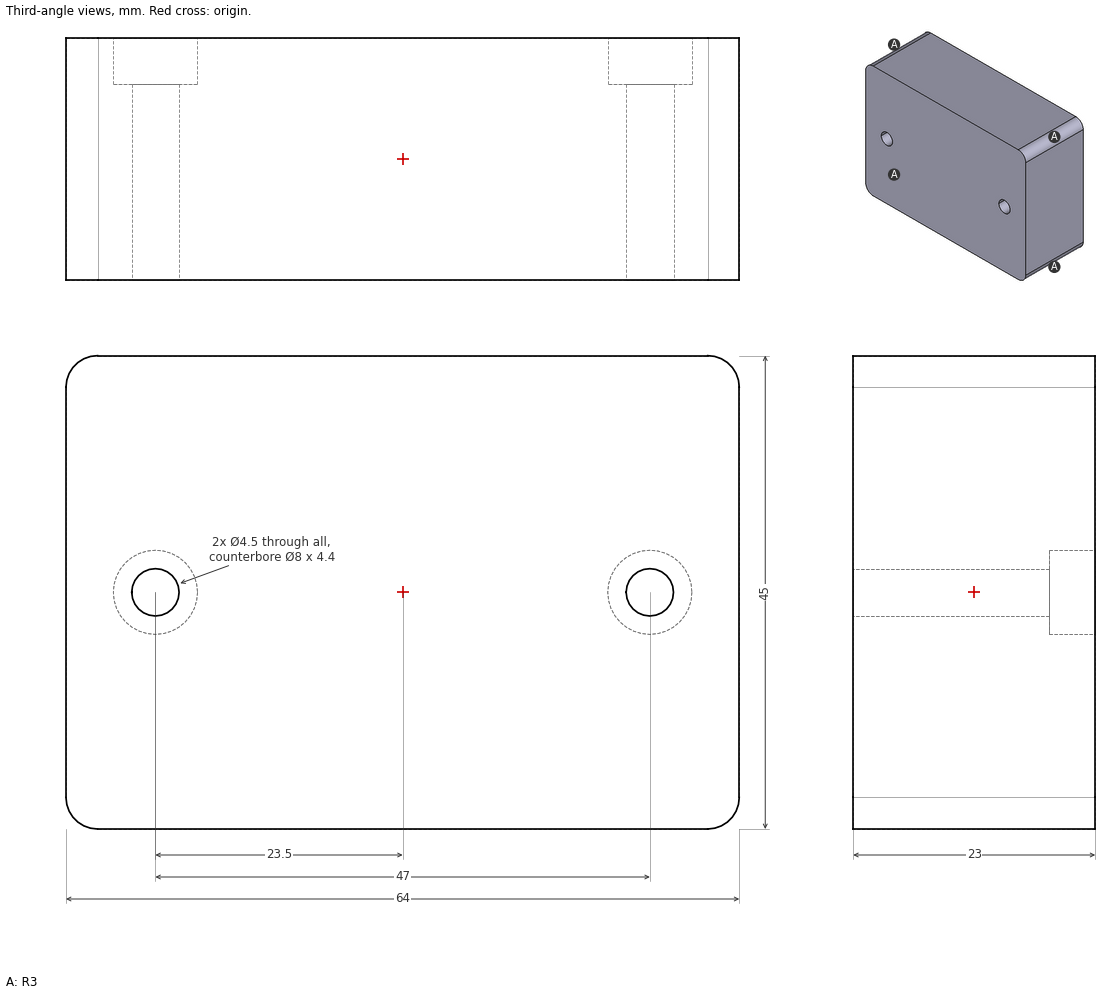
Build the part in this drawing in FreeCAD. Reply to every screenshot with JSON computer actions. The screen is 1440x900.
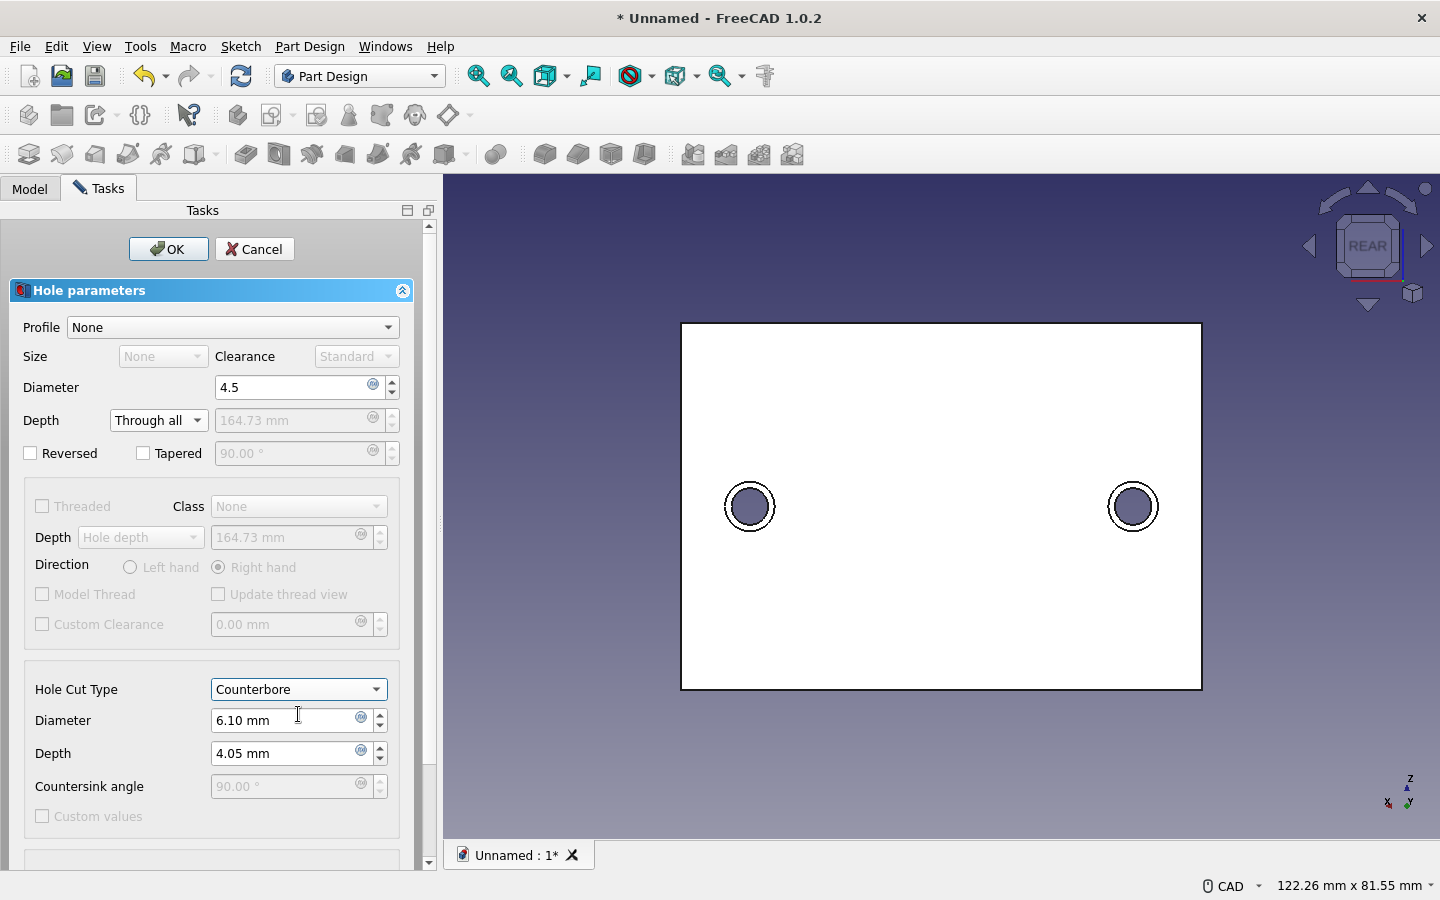
{"action": "triple_click", "coordinate": [292, 720]}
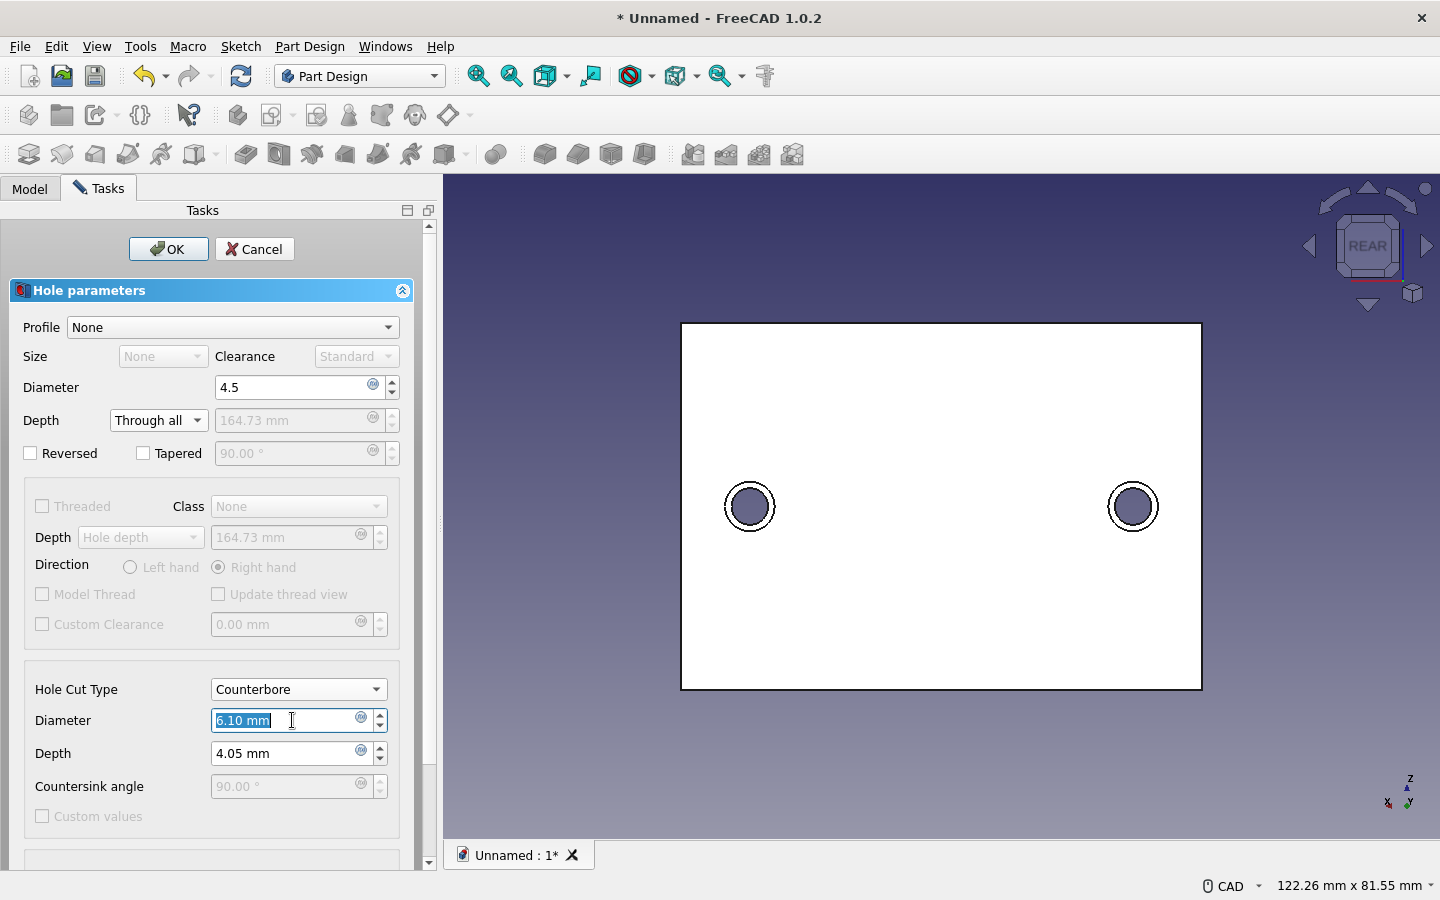
{"action": "type", "text": "8"}
{"action": "key", "text": "Tab"}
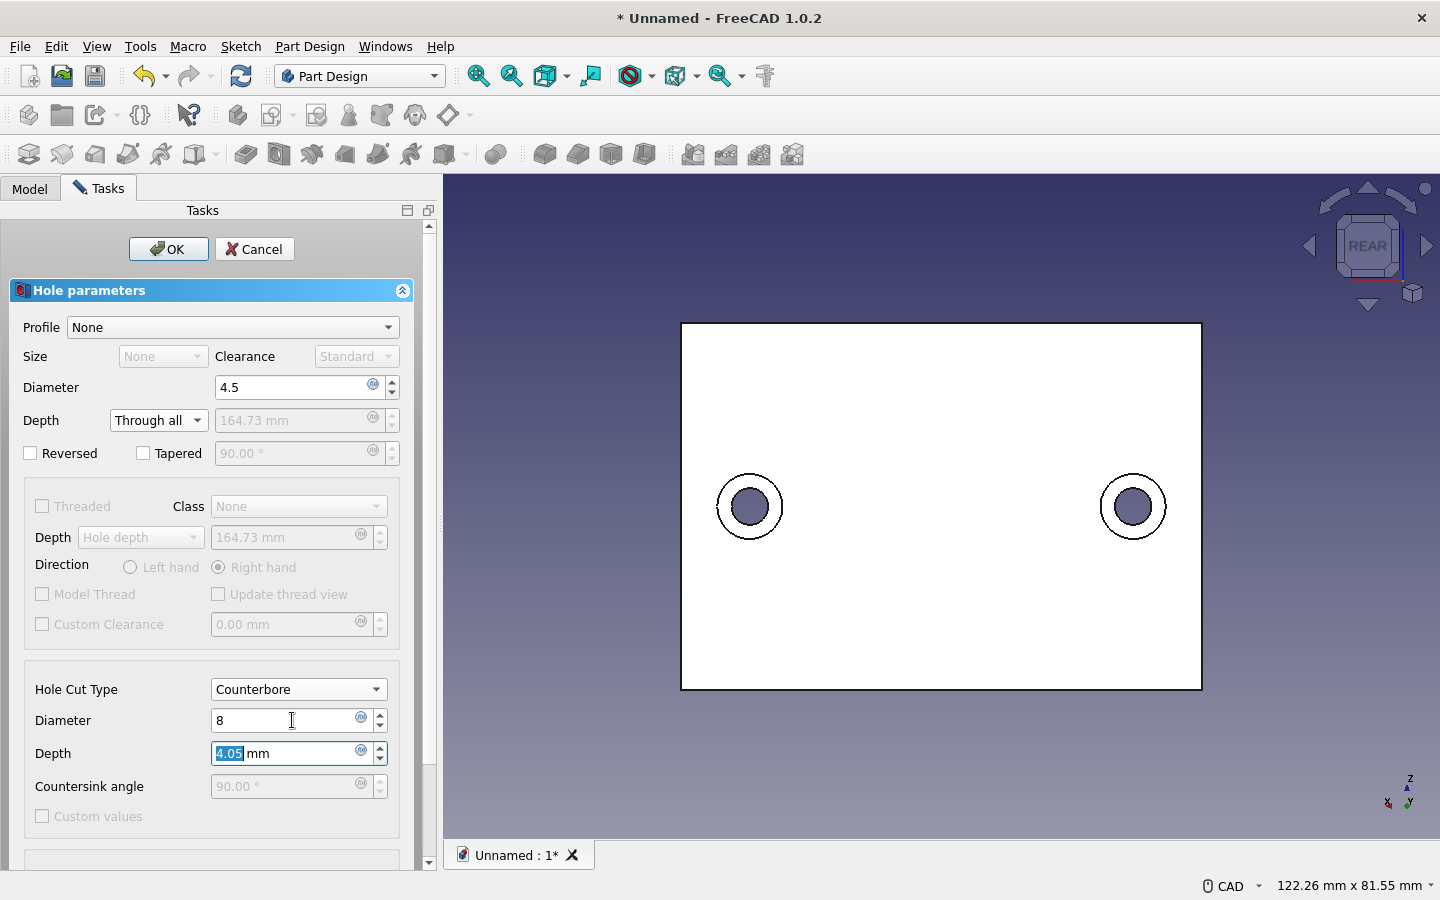
{"action": "type", "text": "4.4"}
{"action": "key", "text": "Tab"}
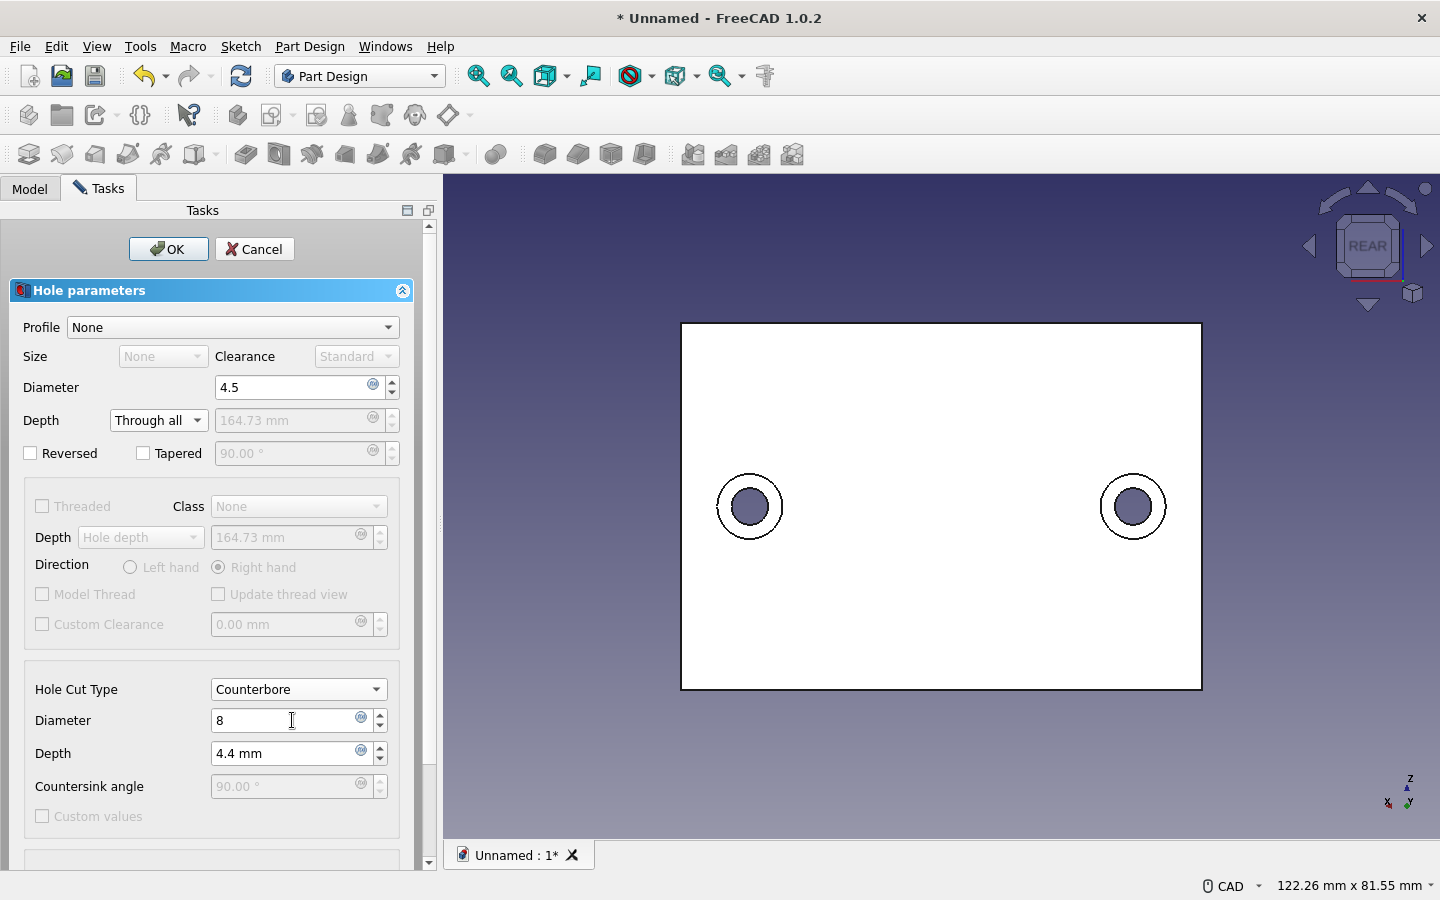
{"action": "left_click", "coordinate": [169, 249]}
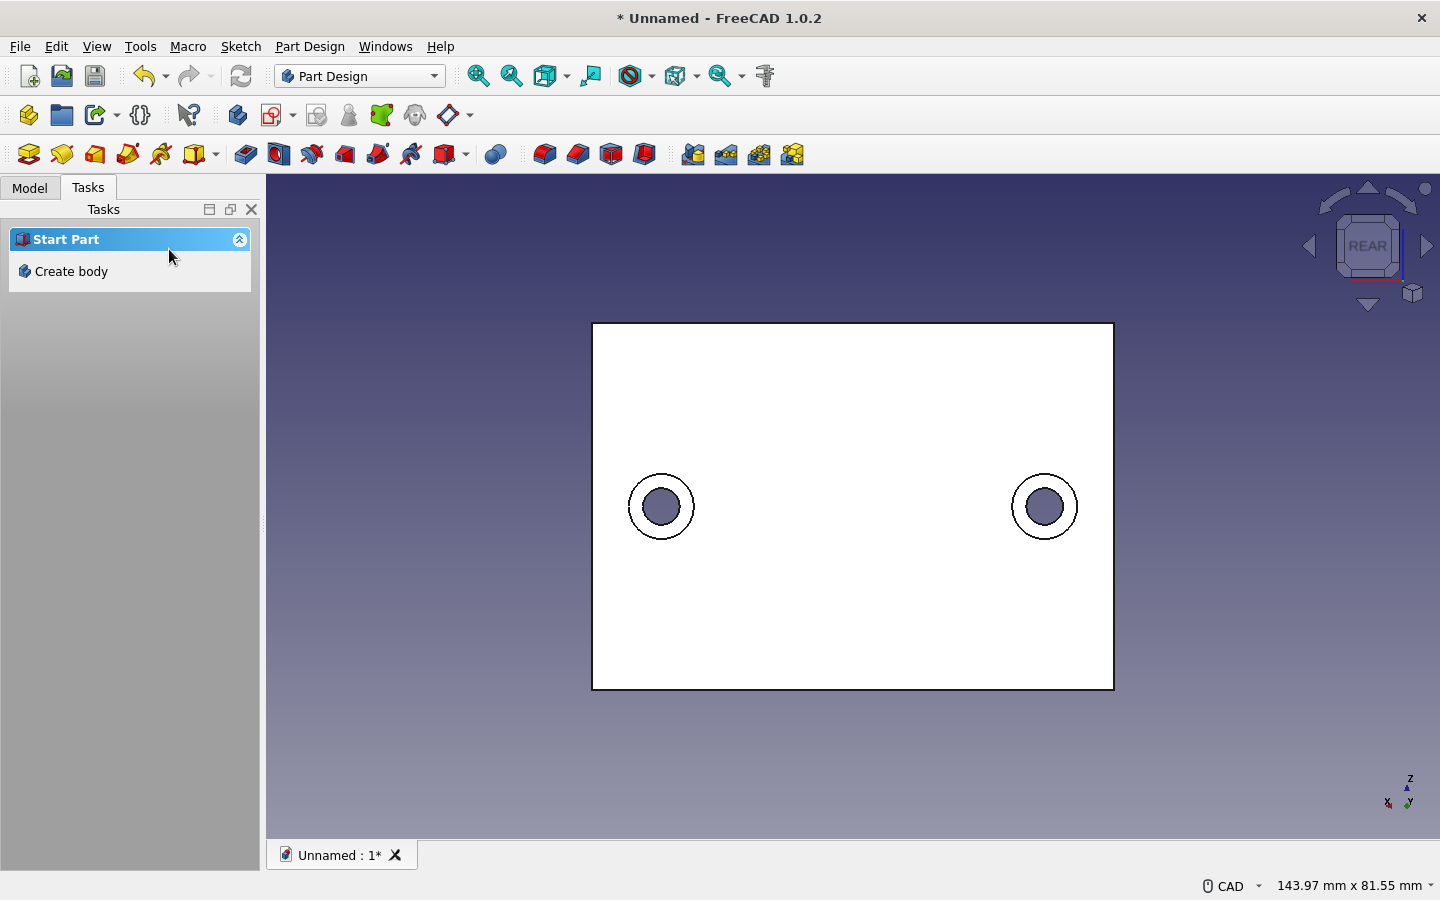
{"action": "key", "text": "0"}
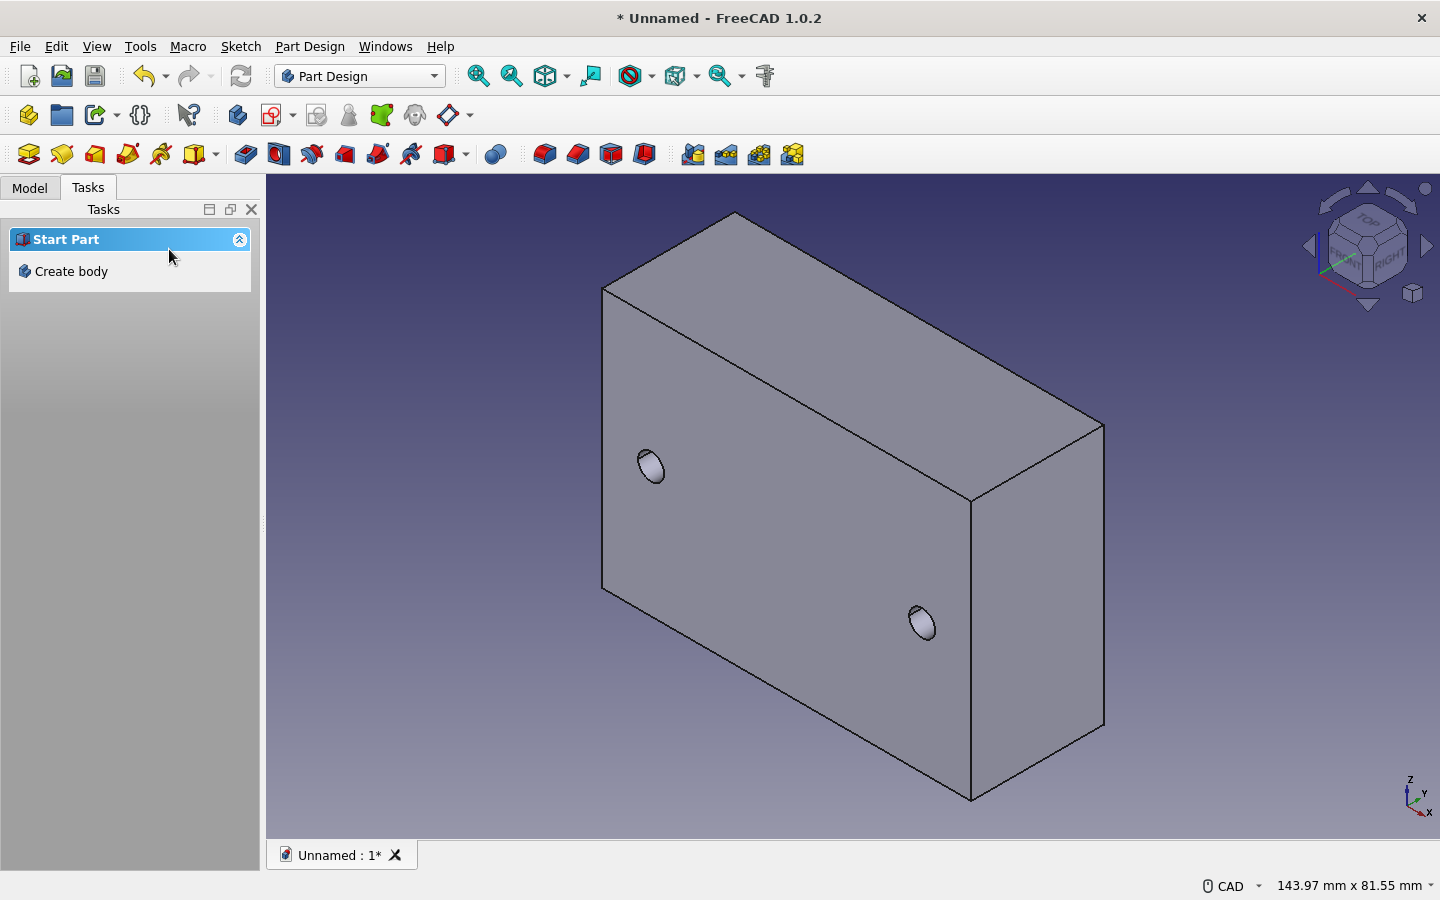
{"action": "left_click", "coordinate": [1038, 462]}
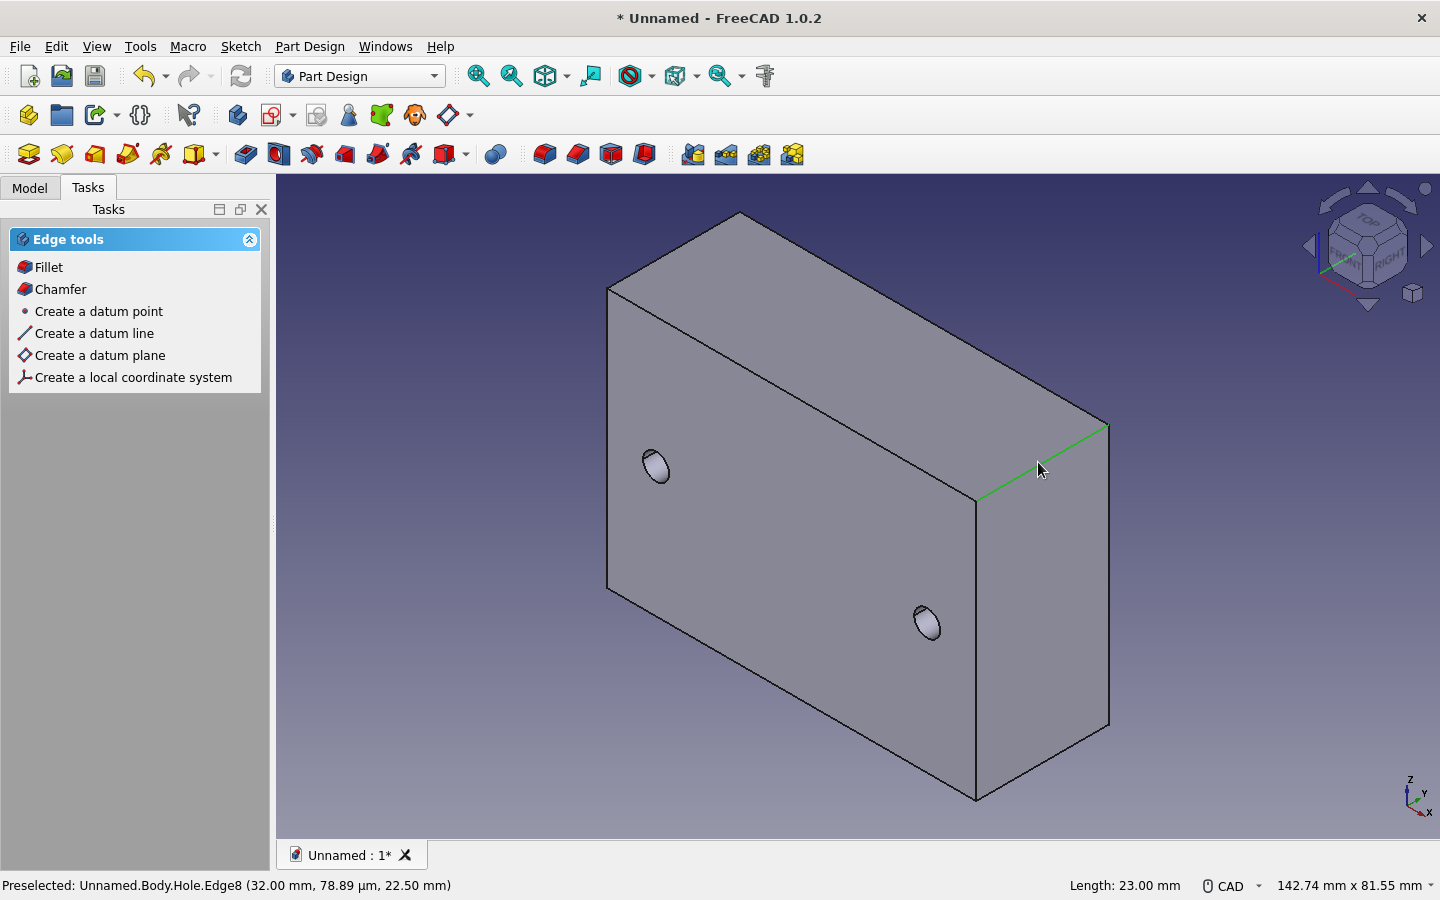
{"action": "key", "text": "2"}